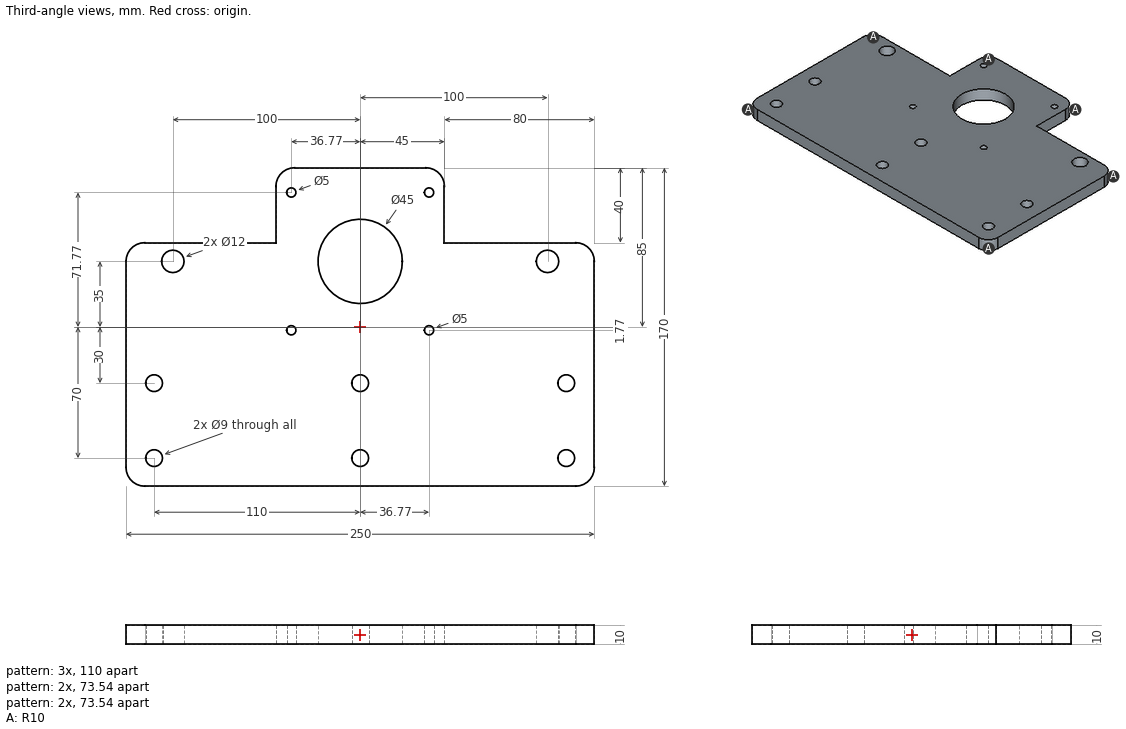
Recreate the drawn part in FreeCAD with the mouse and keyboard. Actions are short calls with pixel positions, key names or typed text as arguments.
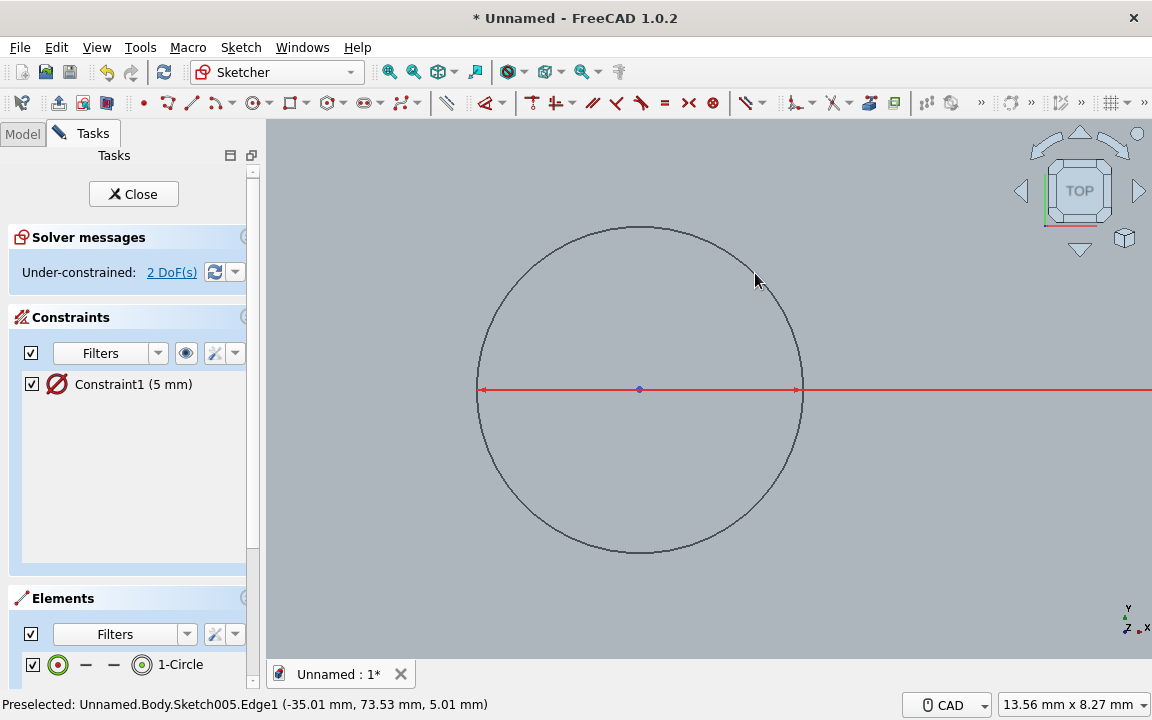
click(486, 104)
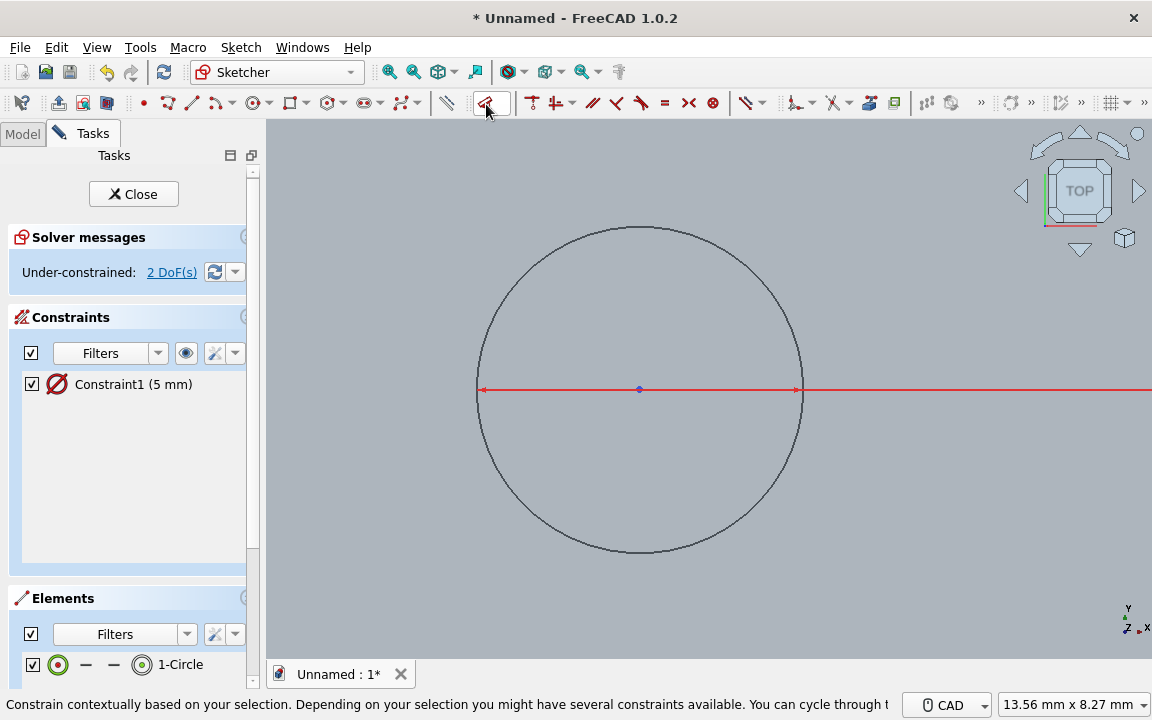
click(640, 390)
click(813, 356)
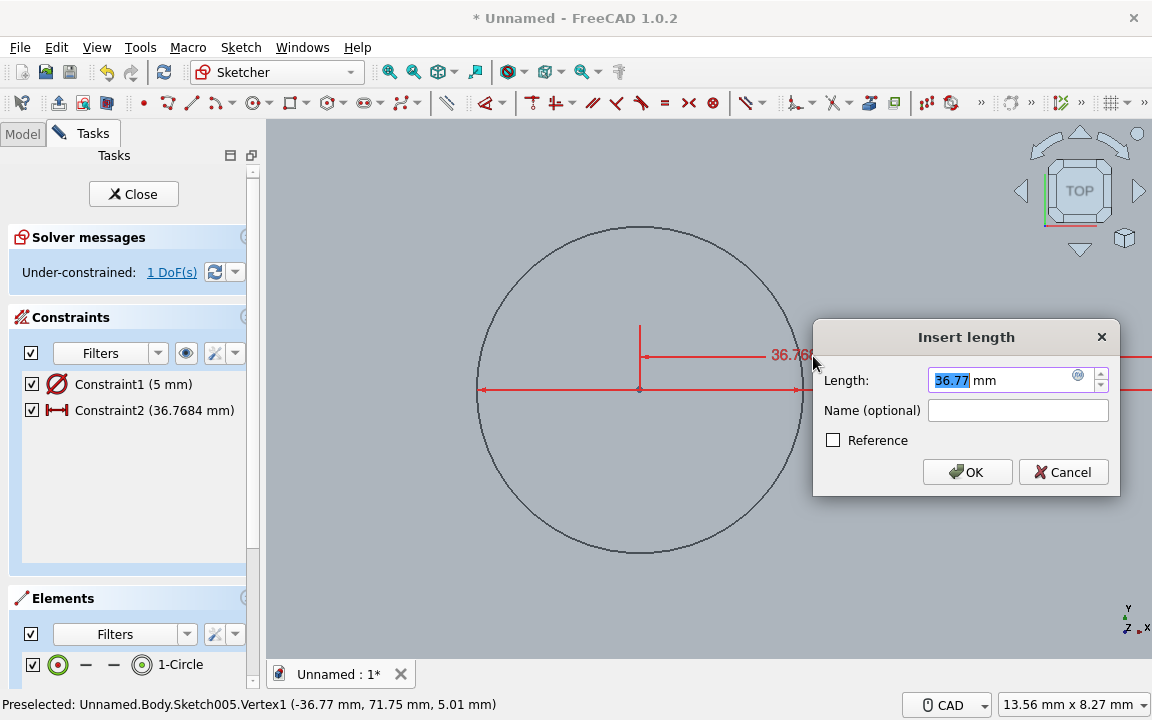
text(36.77)
key(Return)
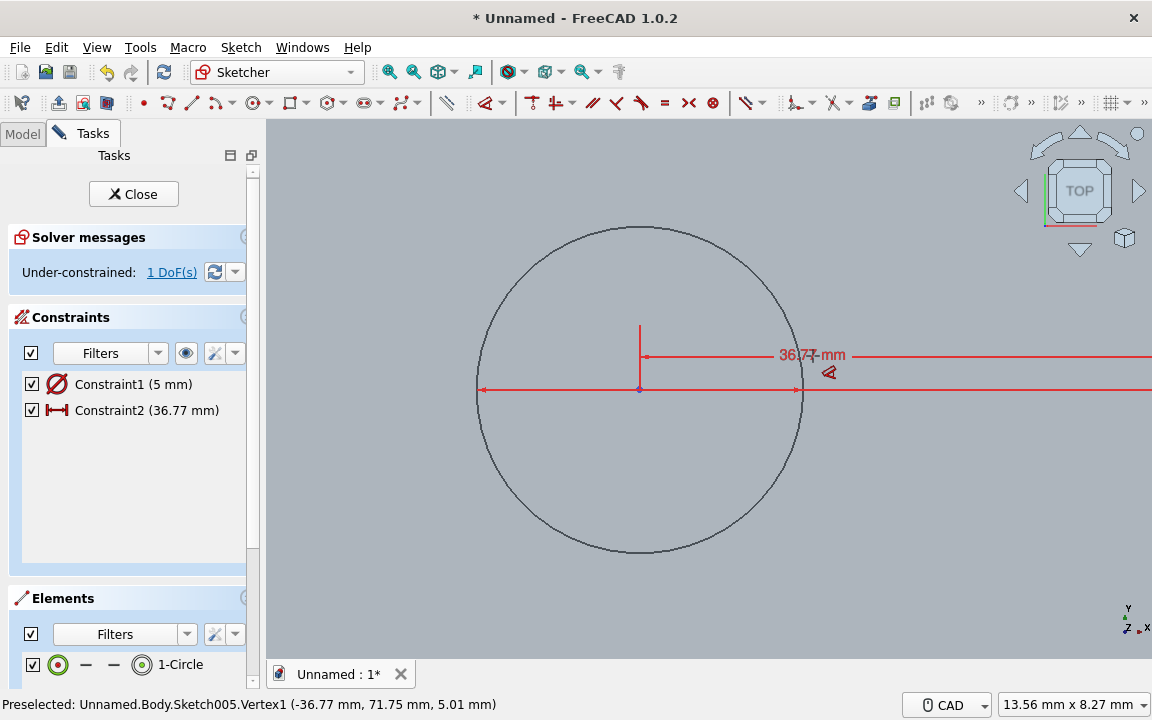
click(640, 390)
click(606, 510)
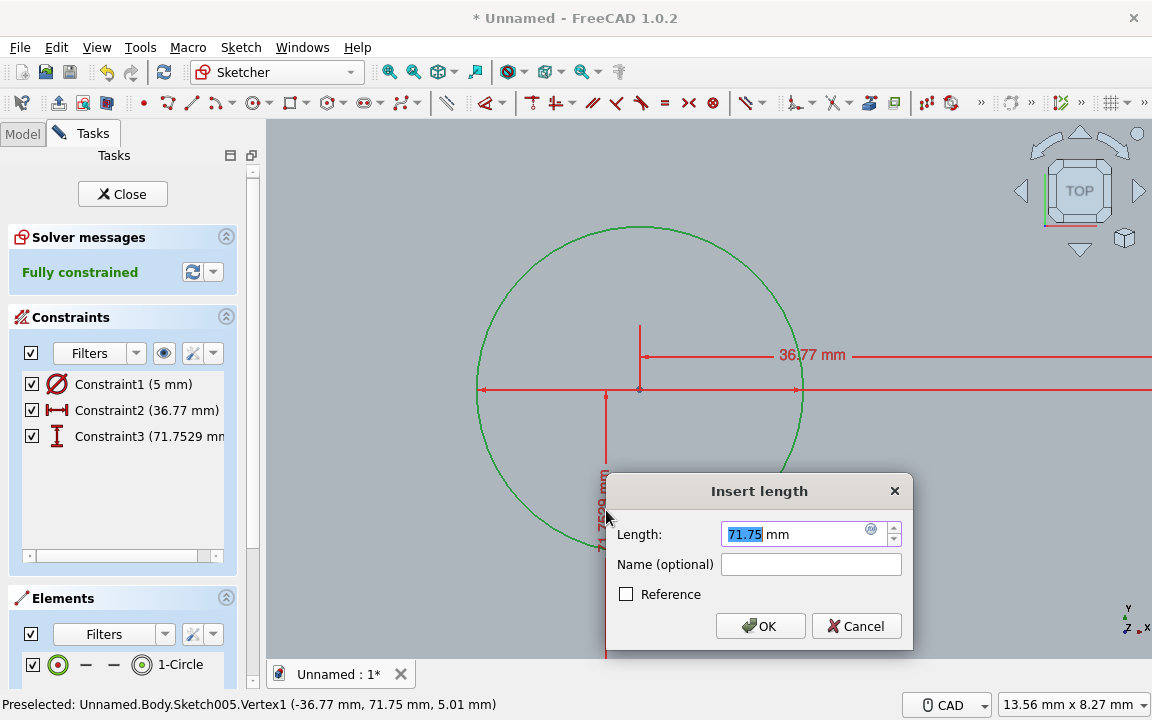
text(71.77)
key(Return)
key(Escape)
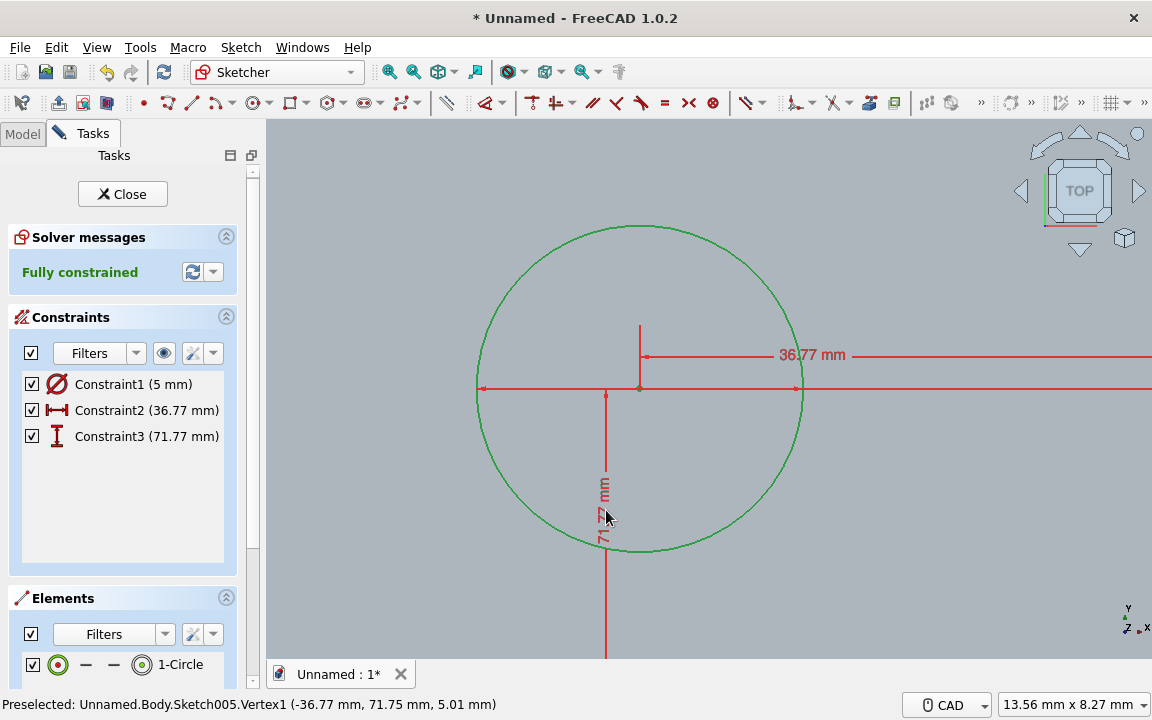
click(123, 194)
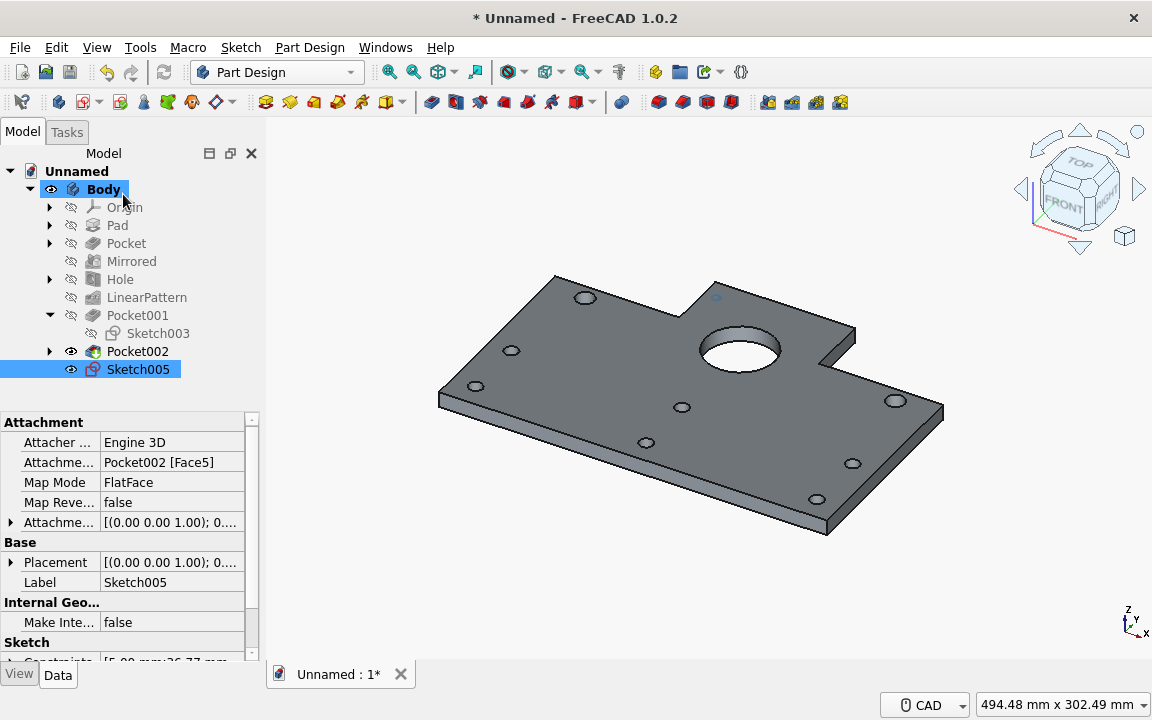
click(432, 102)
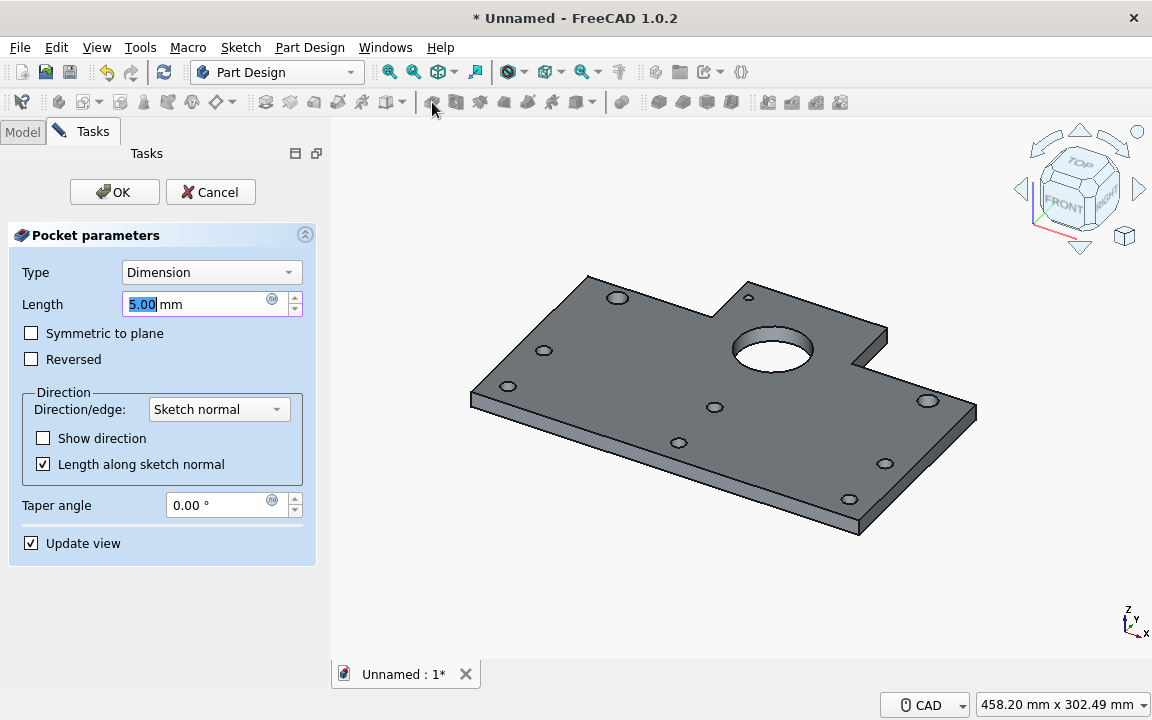
click(212, 272)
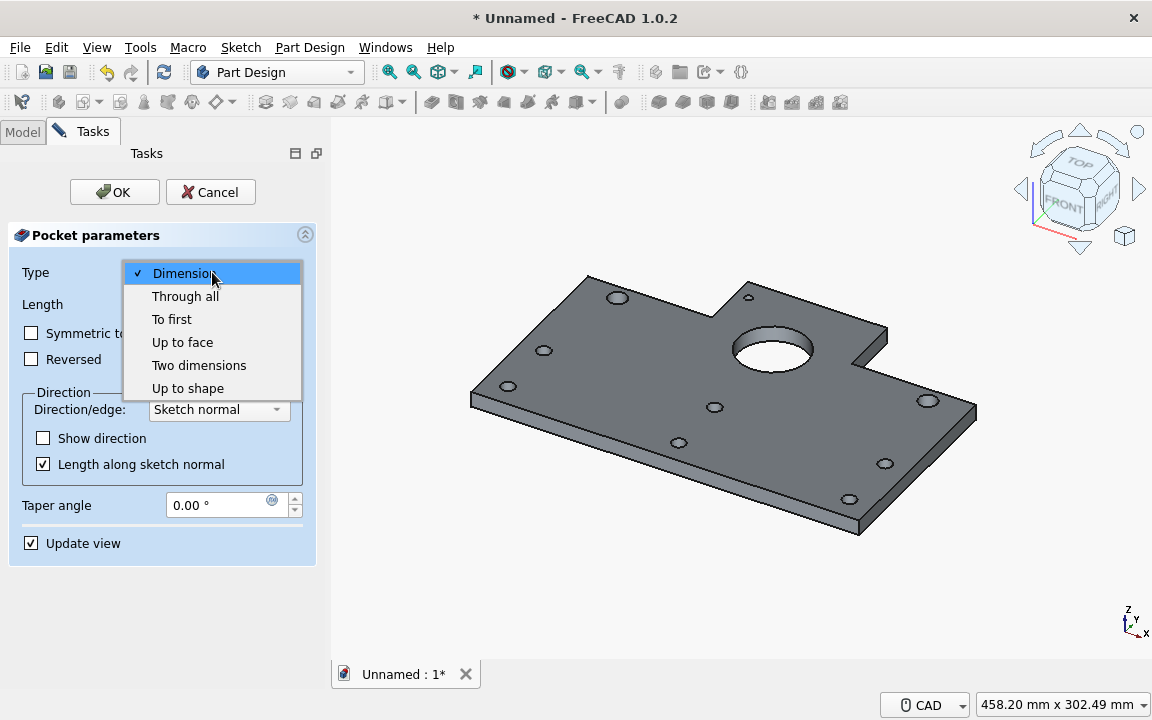
click(212, 296)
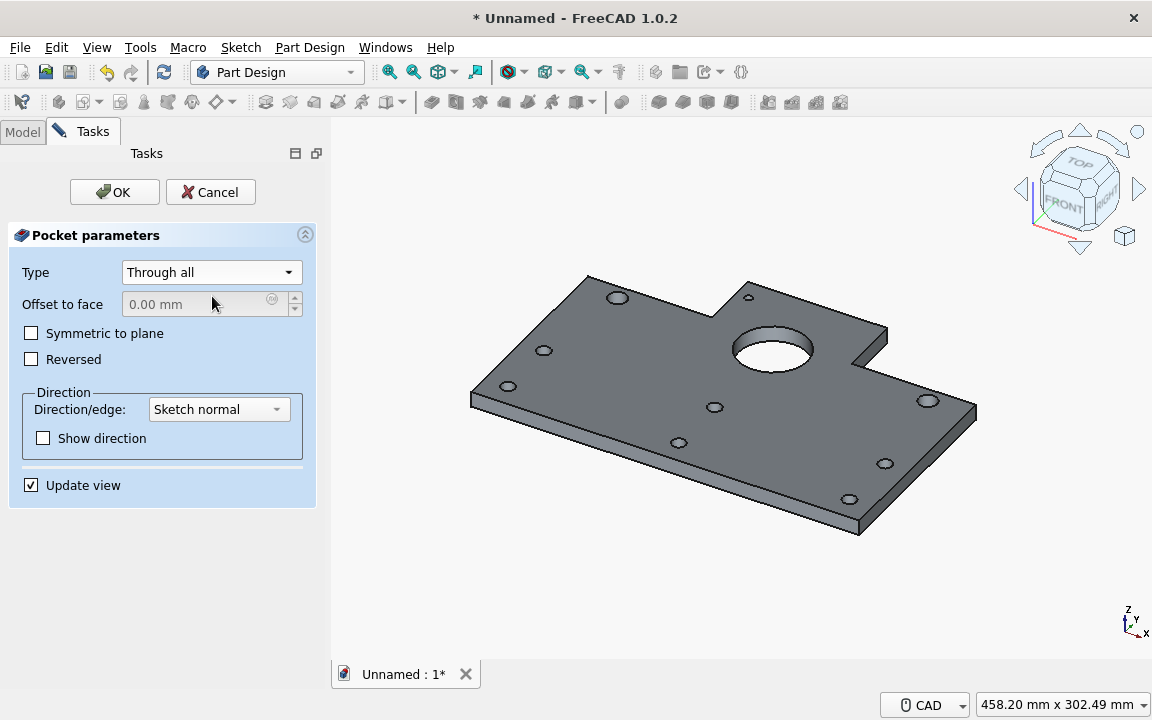
click(115, 192)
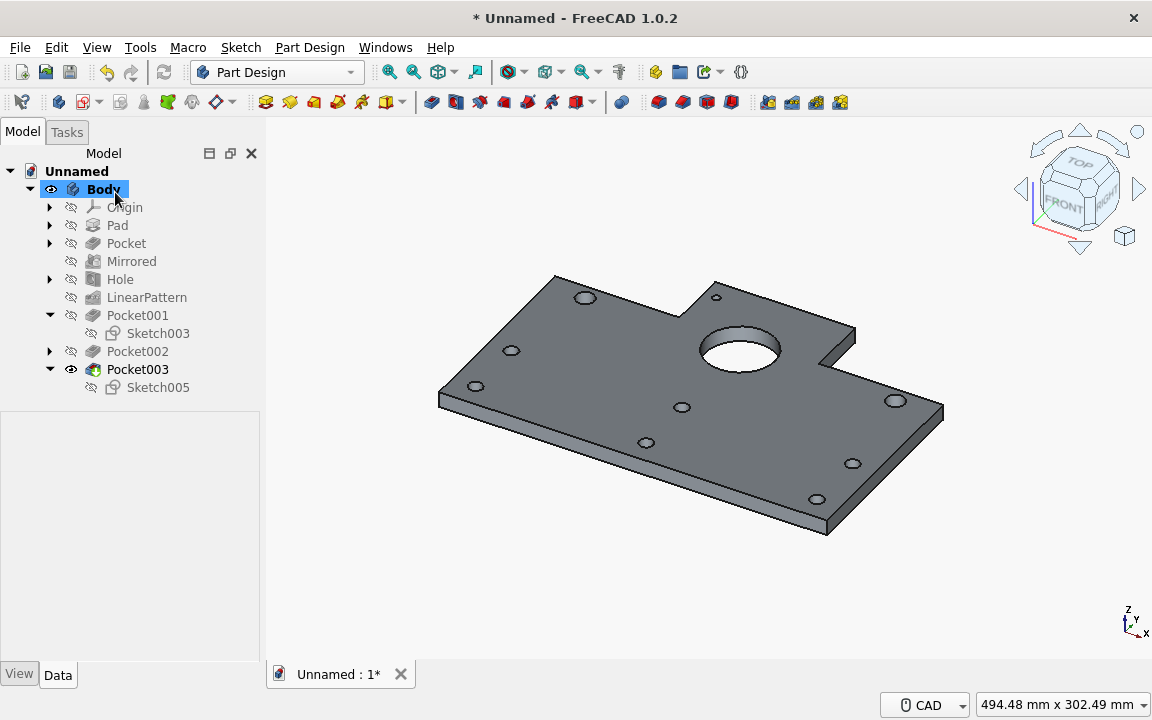
click(116, 369)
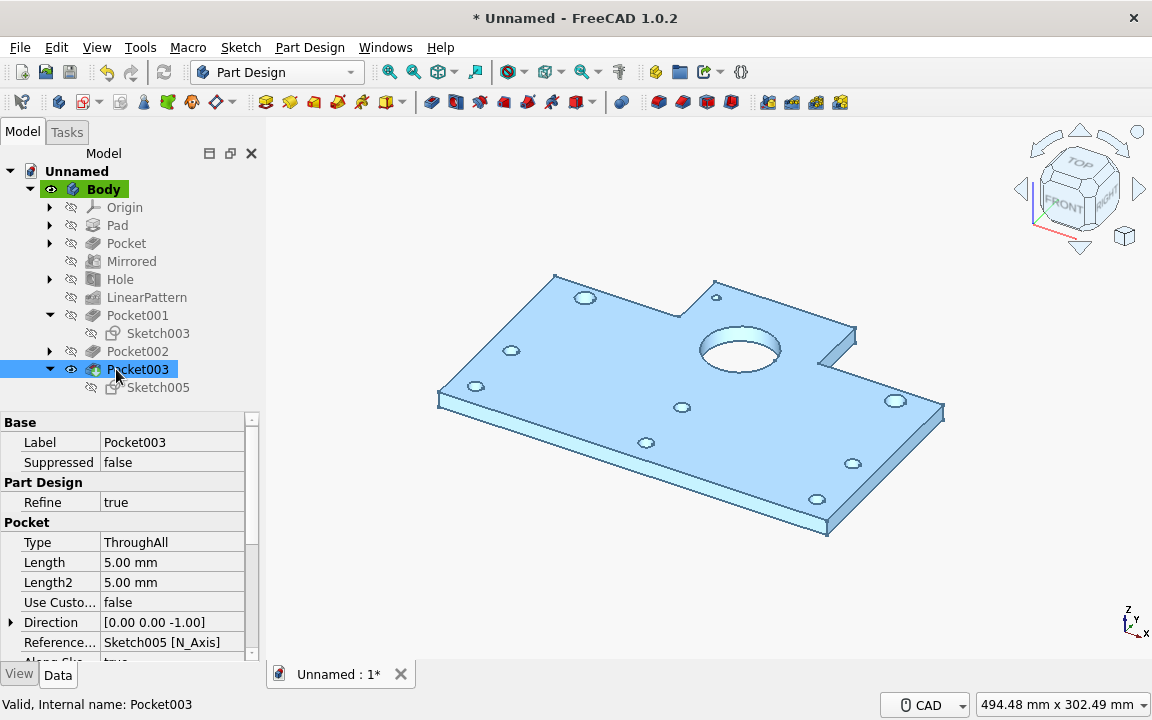
click(792, 102)